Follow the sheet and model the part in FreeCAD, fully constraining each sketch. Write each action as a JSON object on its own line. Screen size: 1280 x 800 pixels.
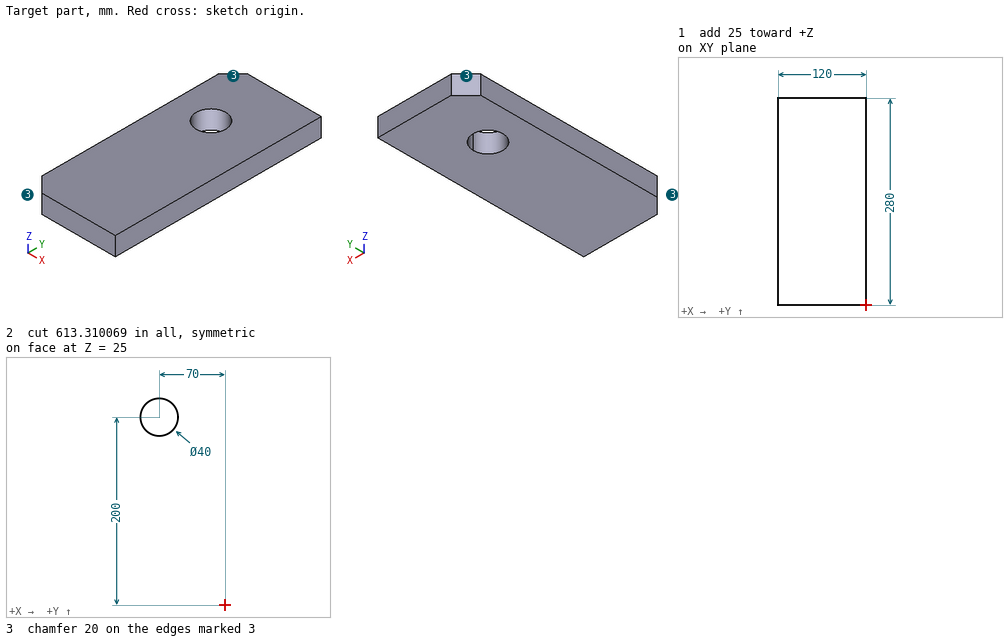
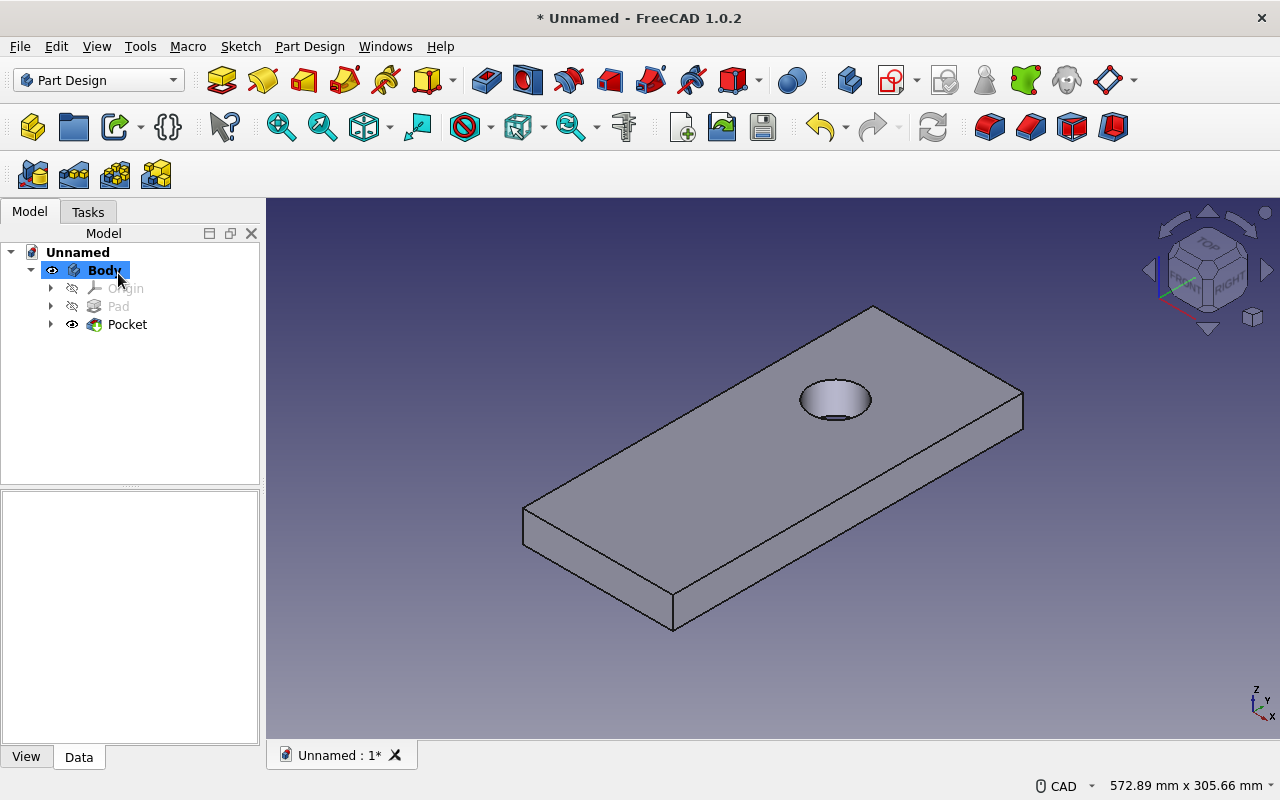
{"action": "key", "text": "2"}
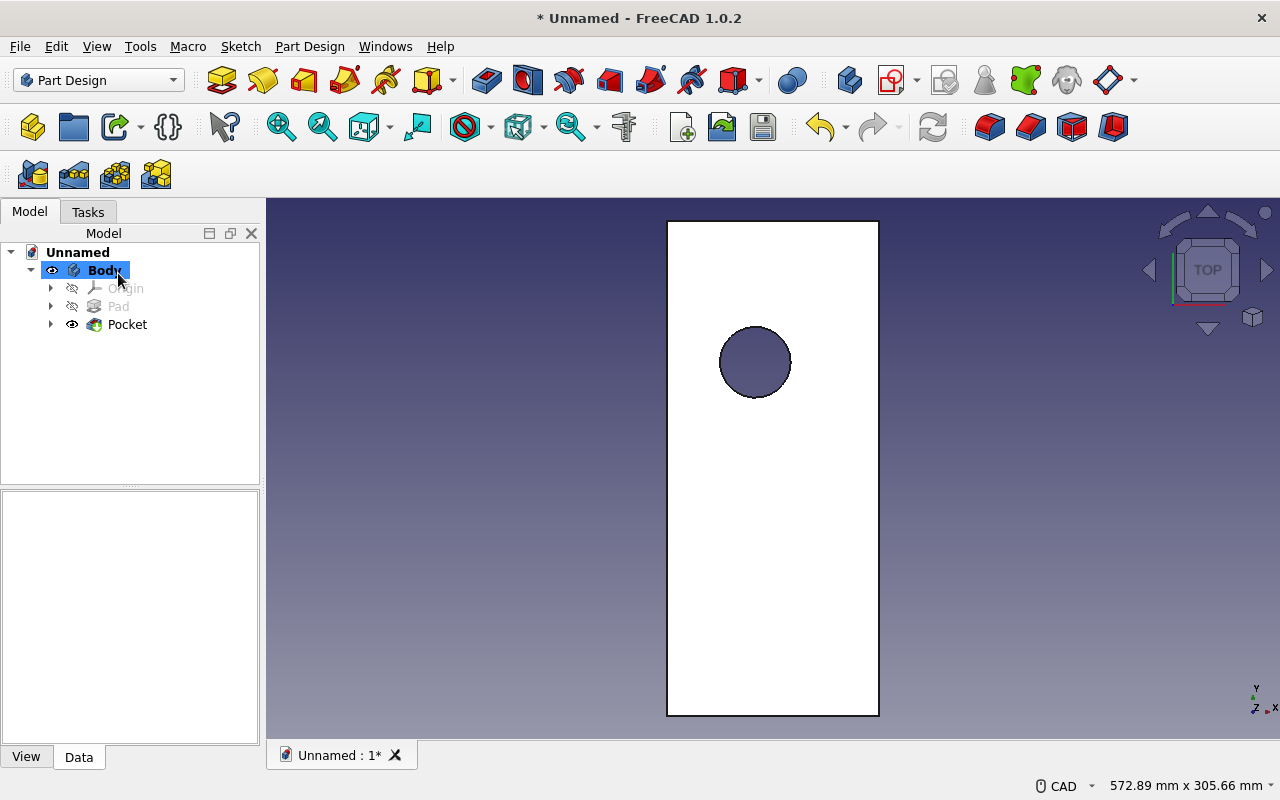
{"action": "key", "text": "1"}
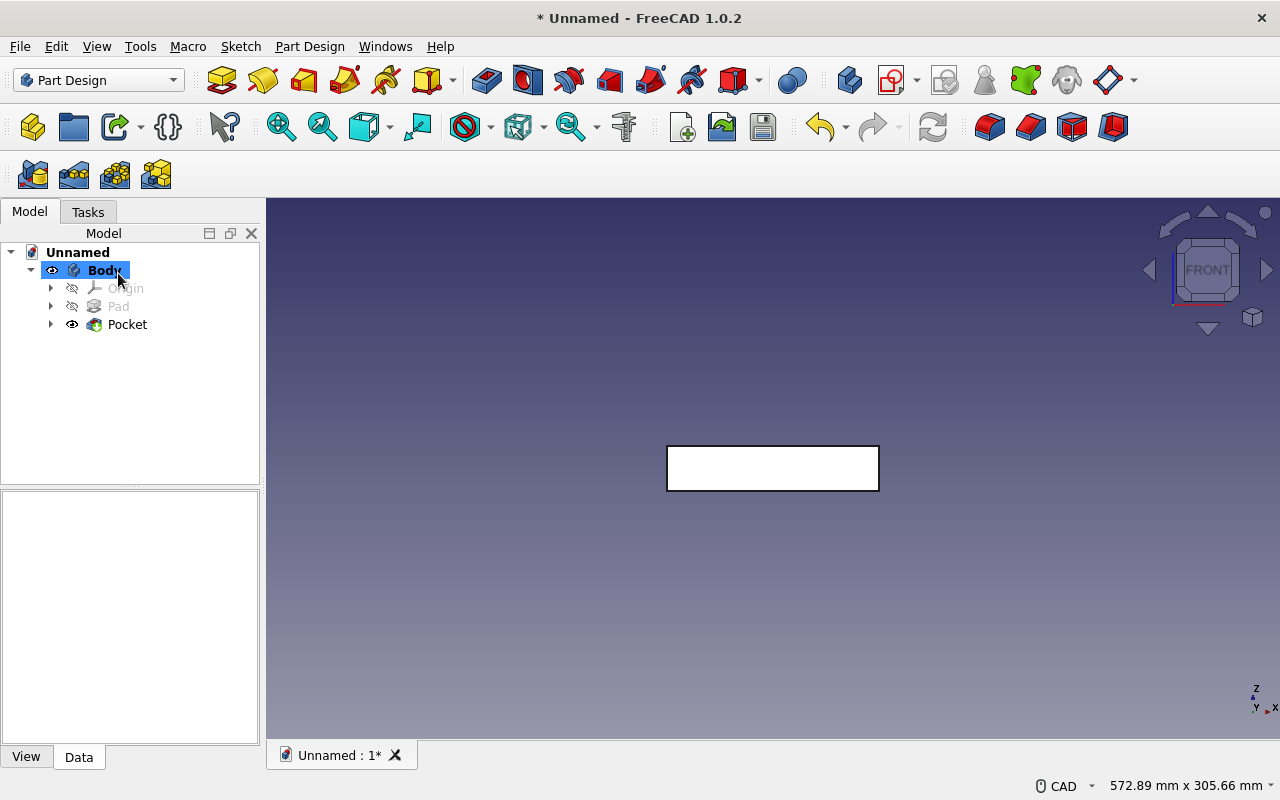
{"action": "left_click", "coordinate": [282, 128]}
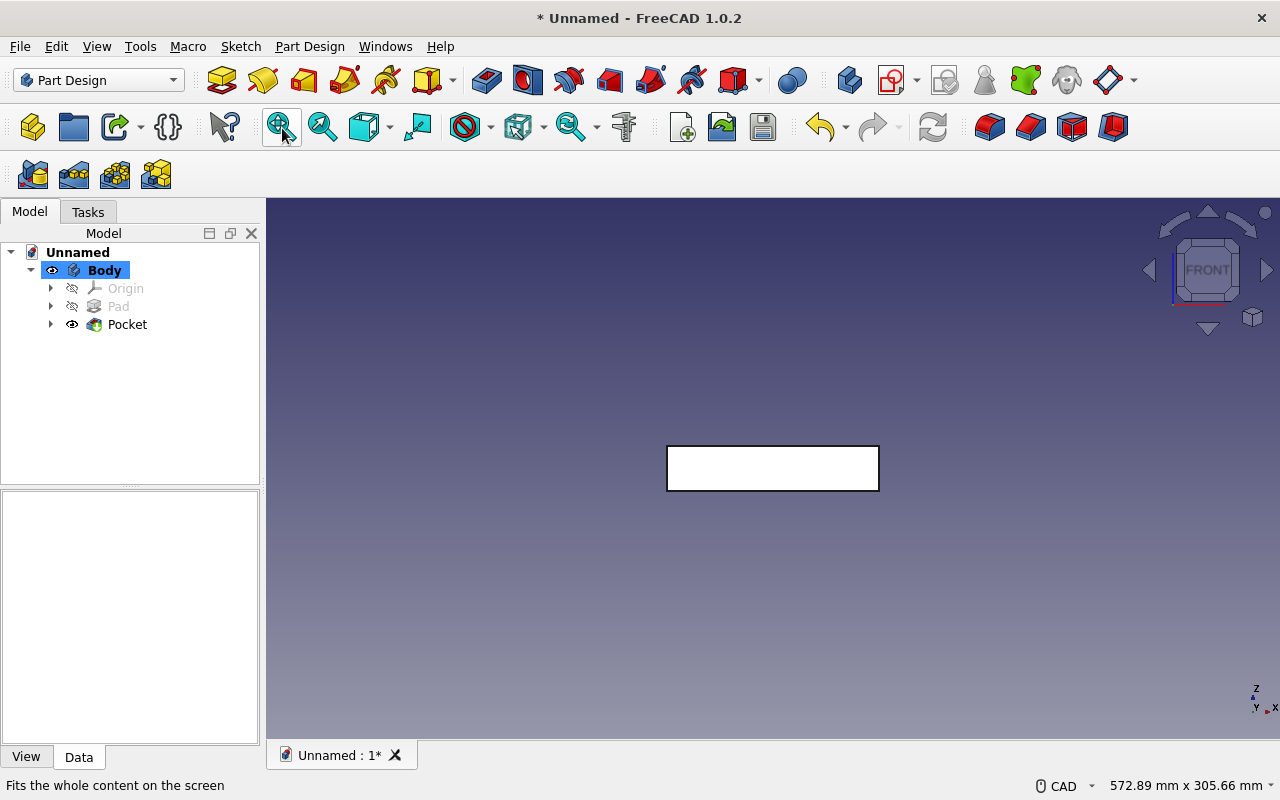
{"action": "left_click", "coordinate": [667, 468]}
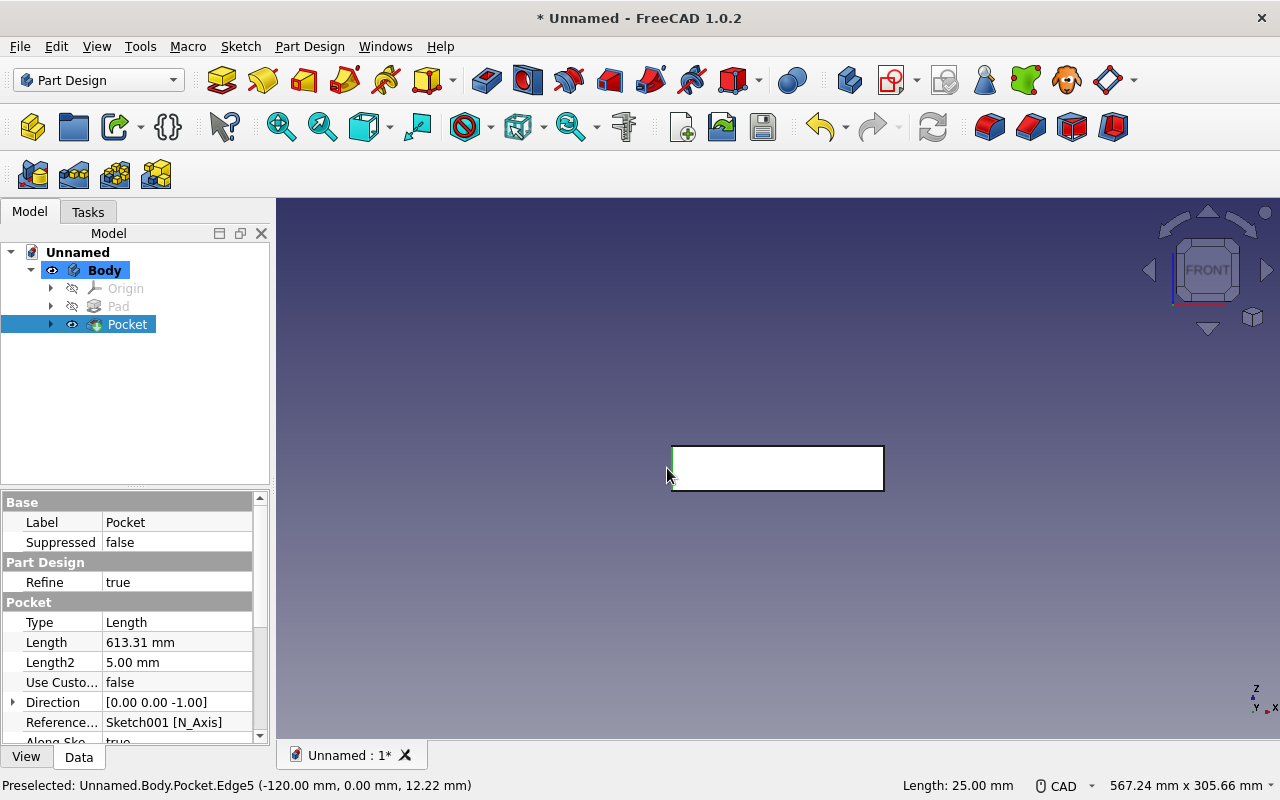
{"action": "key", "text": "3"}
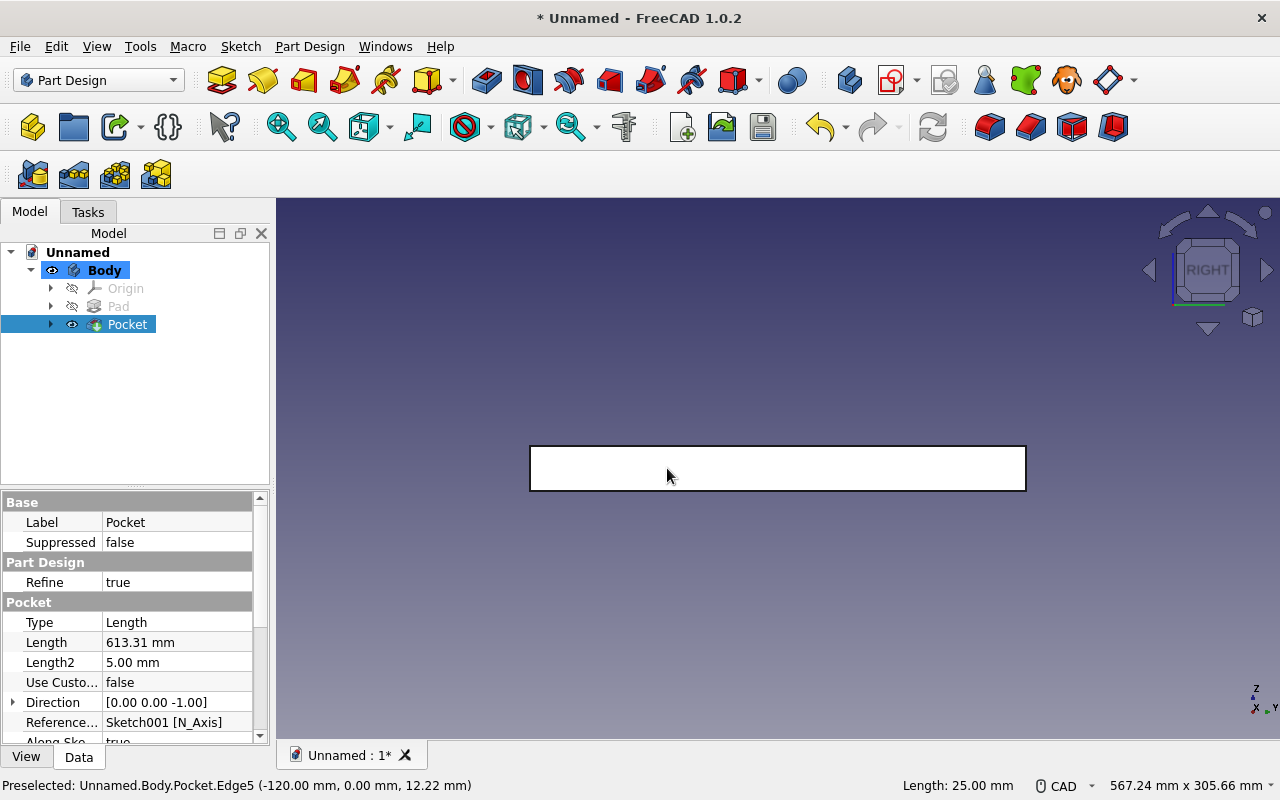
{"action": "key", "text": "5"}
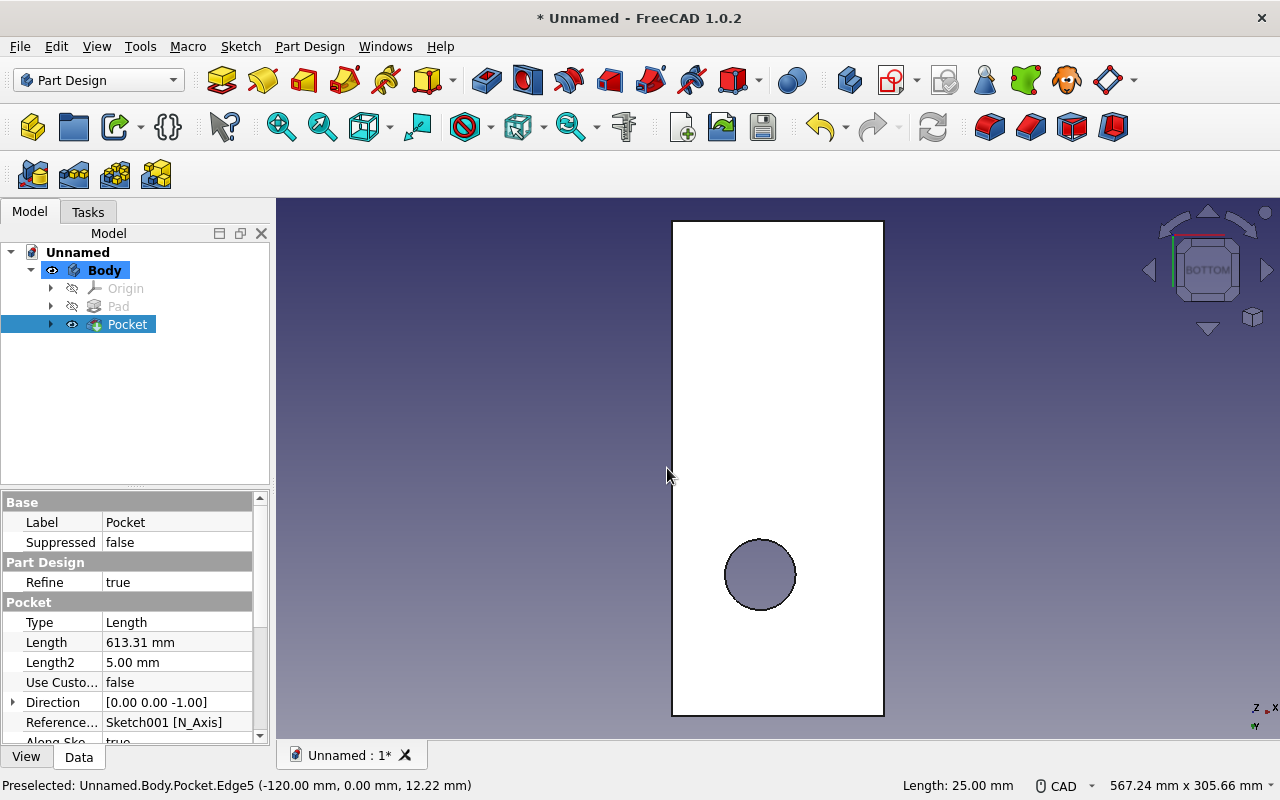
{"action": "key", "text": "4"}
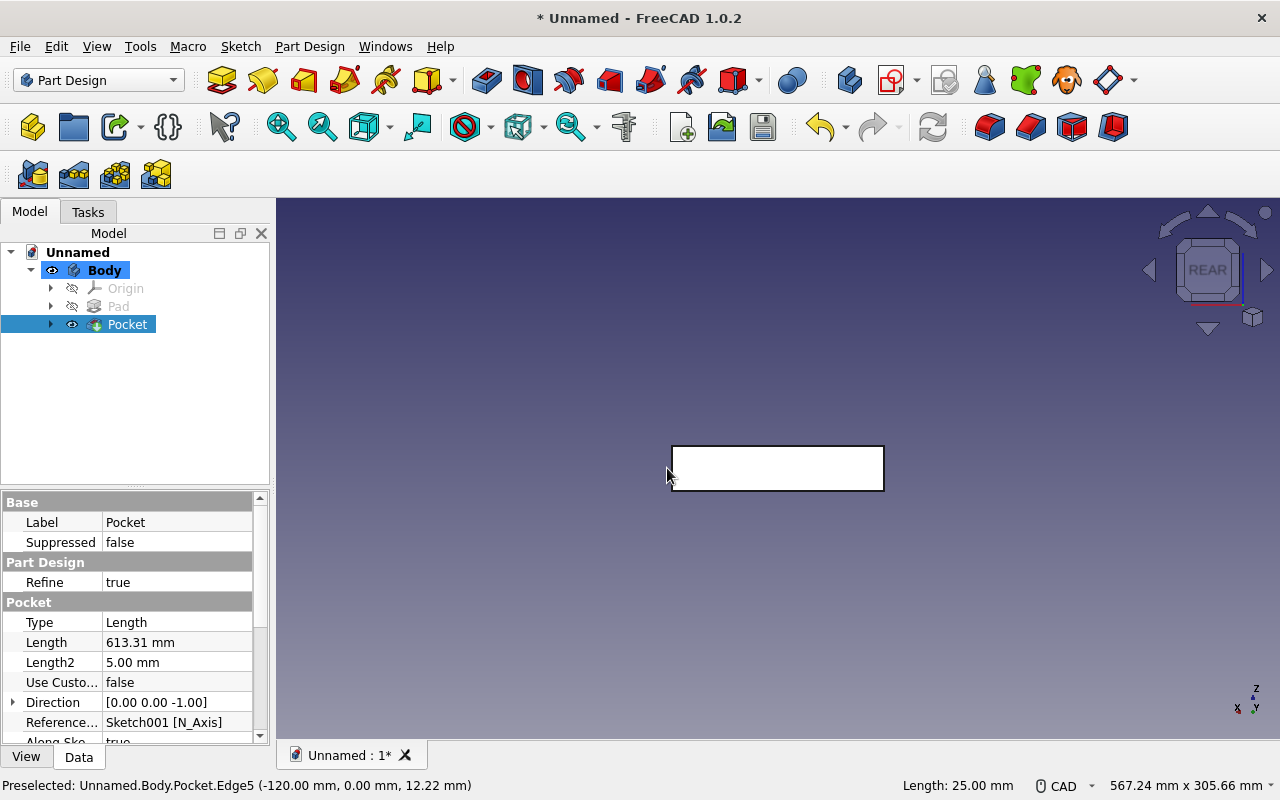
{"action": "left_click", "coordinate": [282, 128]}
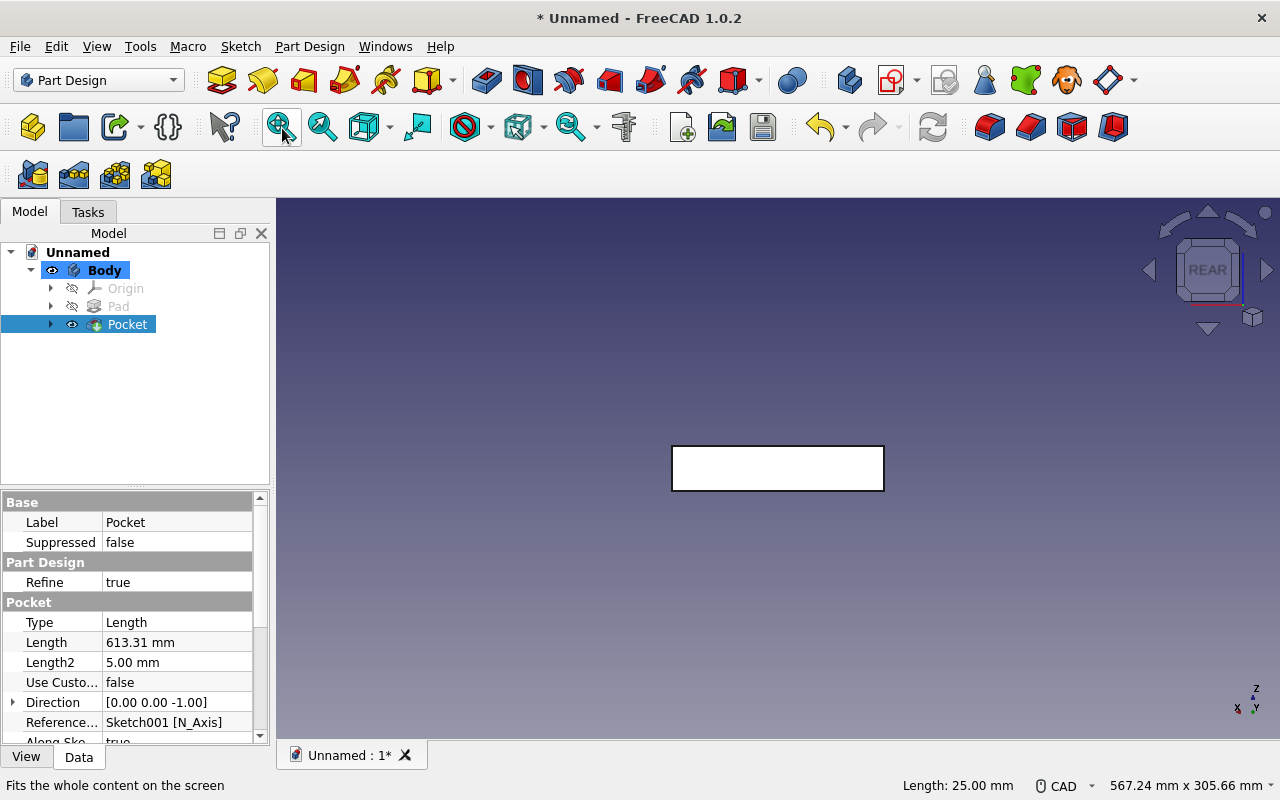
{"action": "left_click", "coordinate": [884, 468], "text": "ctrl"}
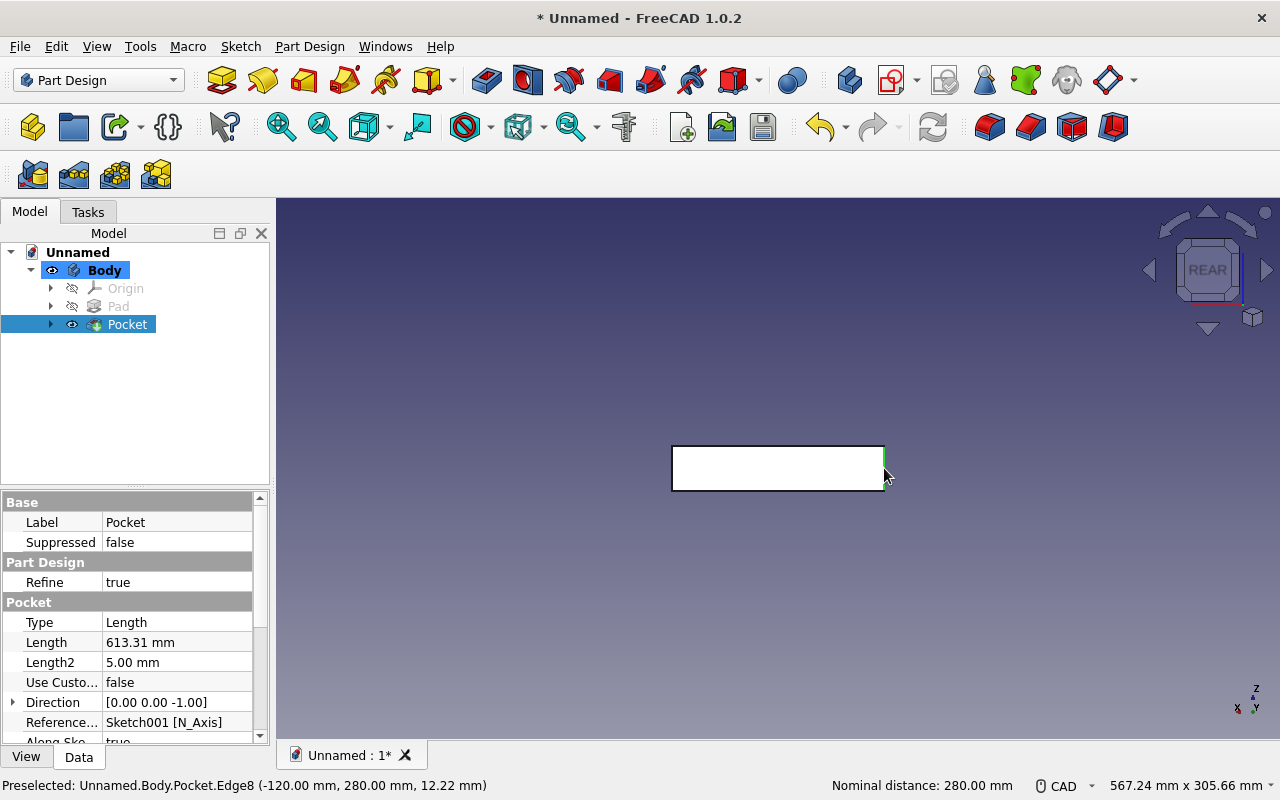
{"action": "left_click", "coordinate": [1031, 128]}